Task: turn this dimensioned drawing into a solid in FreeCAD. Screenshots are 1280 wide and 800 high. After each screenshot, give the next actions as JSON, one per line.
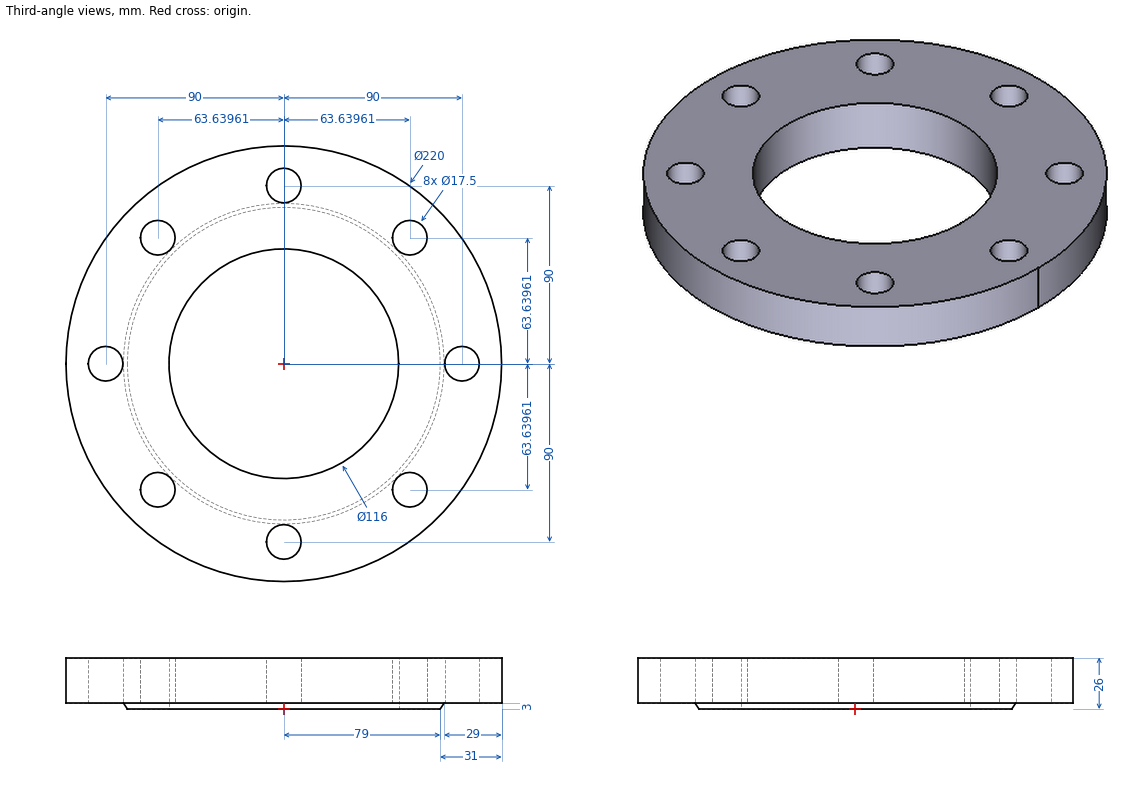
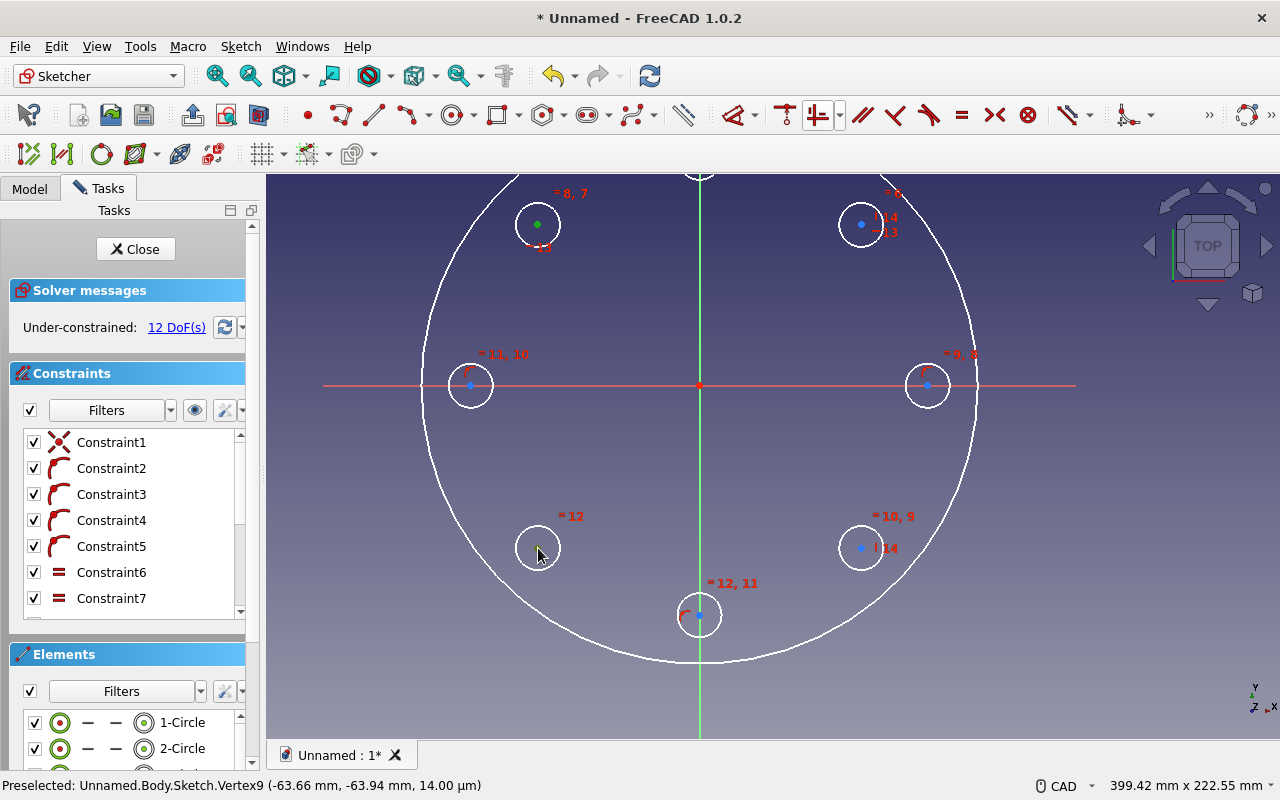
{"action": "left_click", "coordinate": [840, 116]}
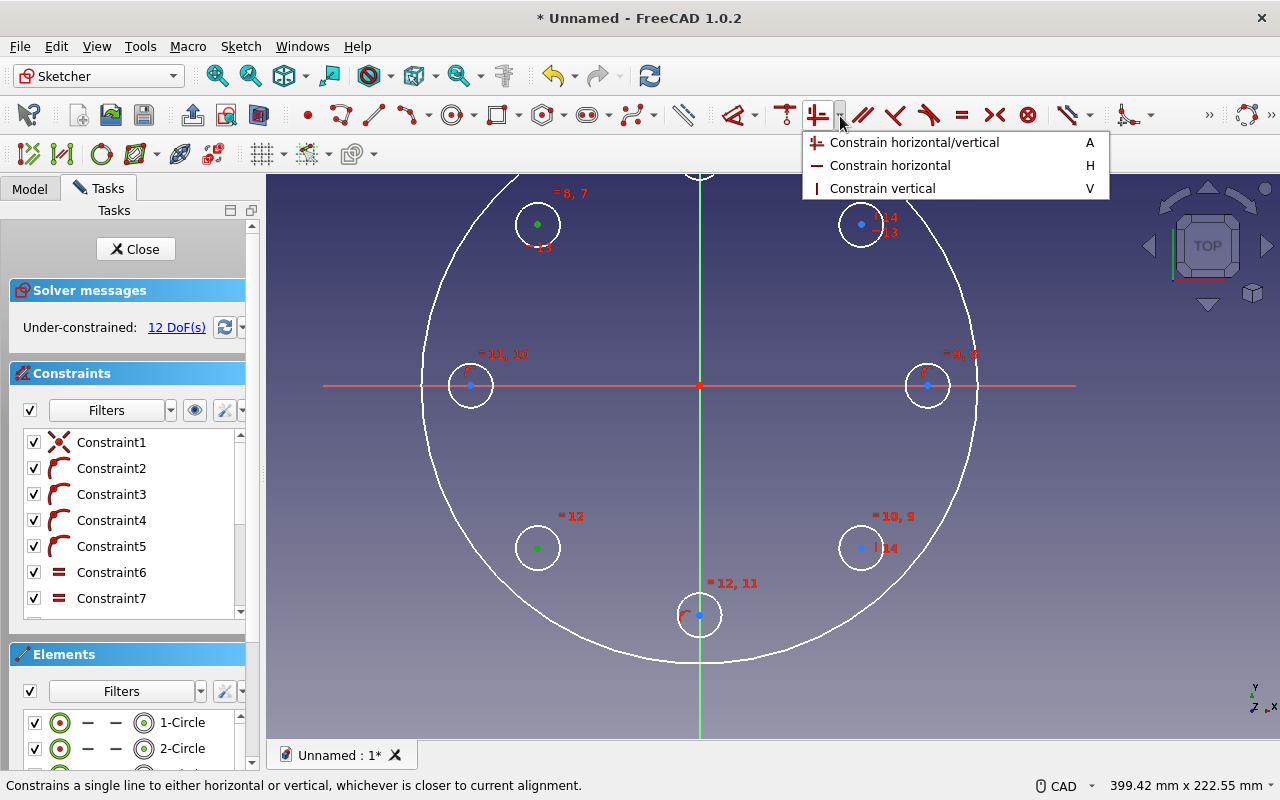
{"action": "left_click", "coordinate": [956, 188]}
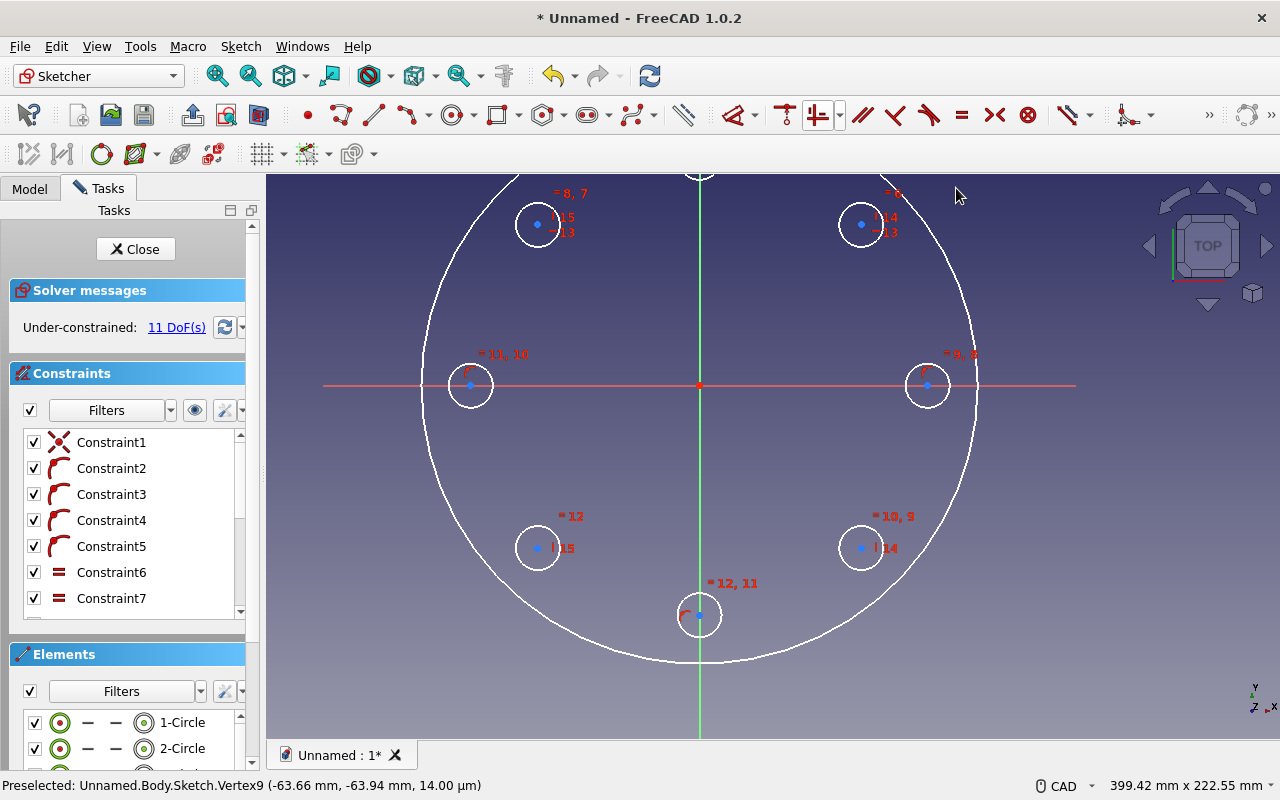
{"action": "left_click", "coordinate": [861, 548]}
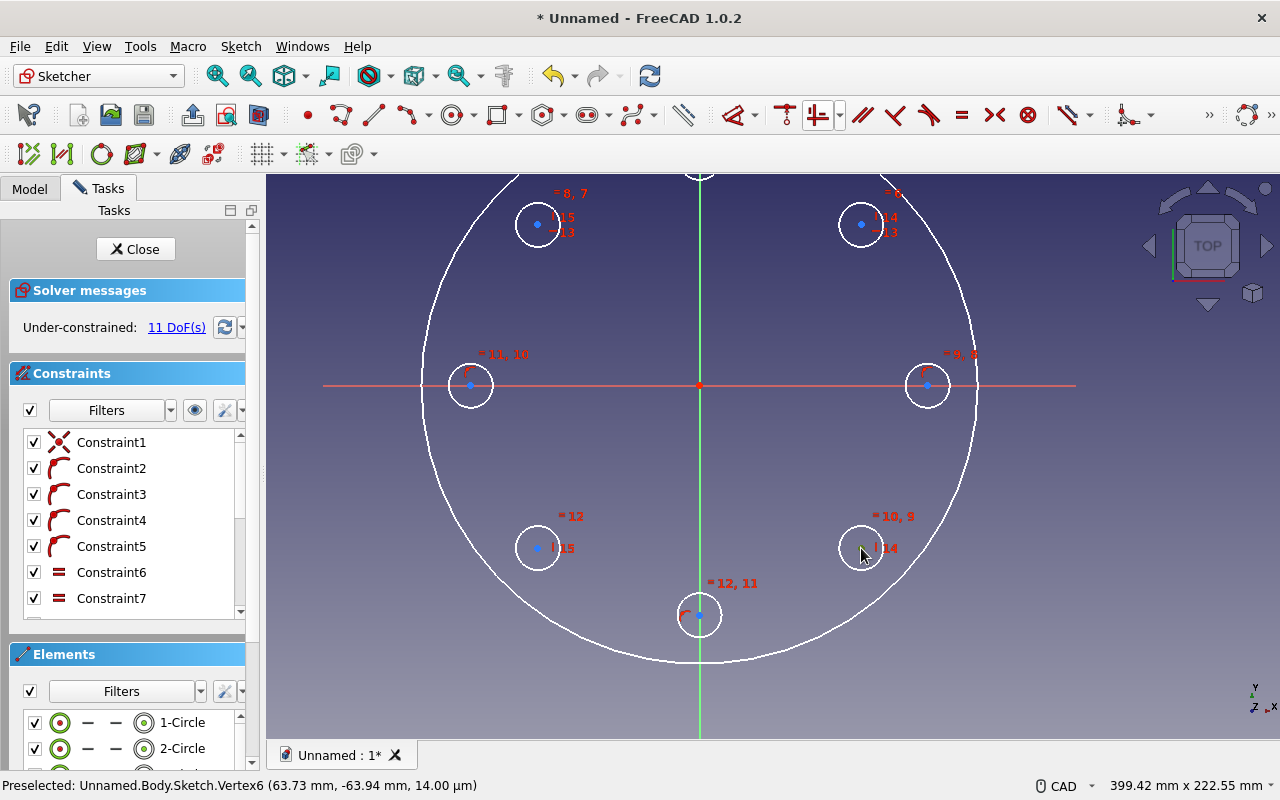
{"action": "left_click", "coordinate": [538, 548]}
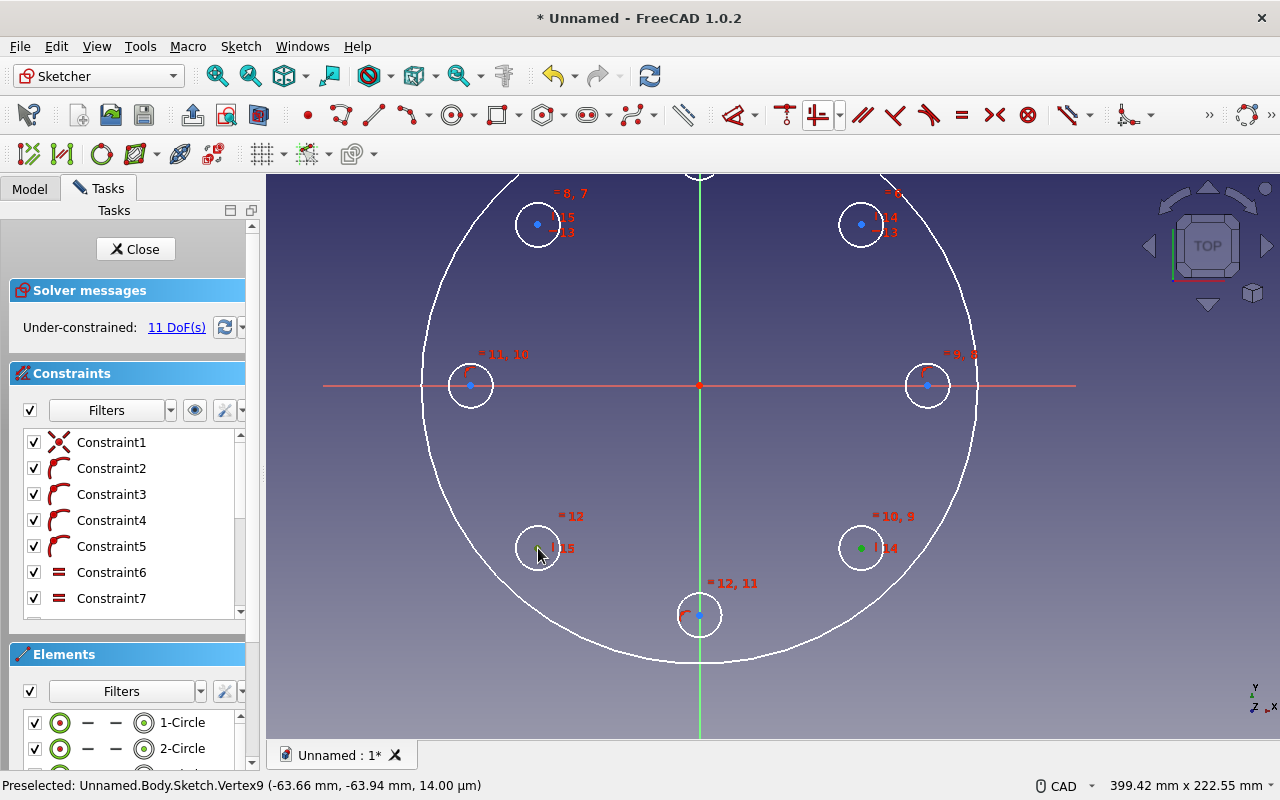
{"action": "left_click", "coordinate": [840, 116]}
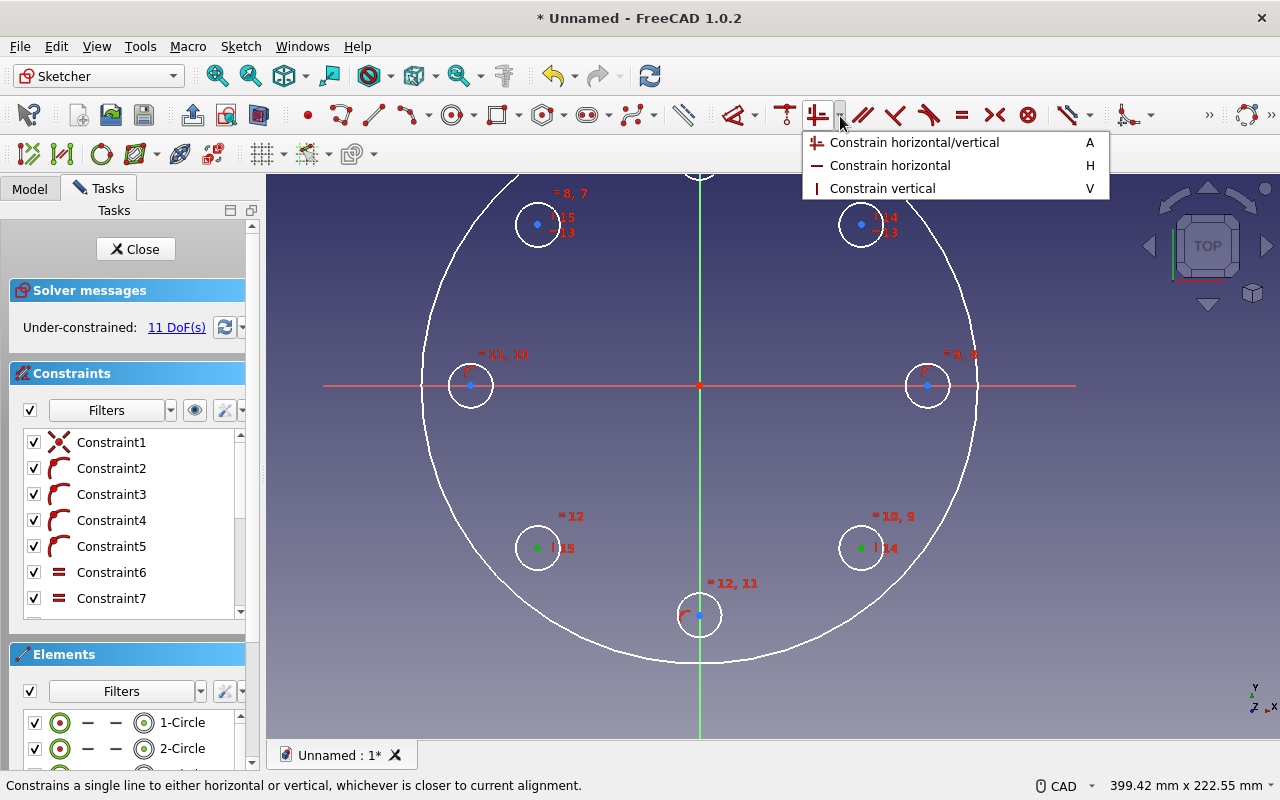
{"action": "left_click", "coordinate": [956, 166]}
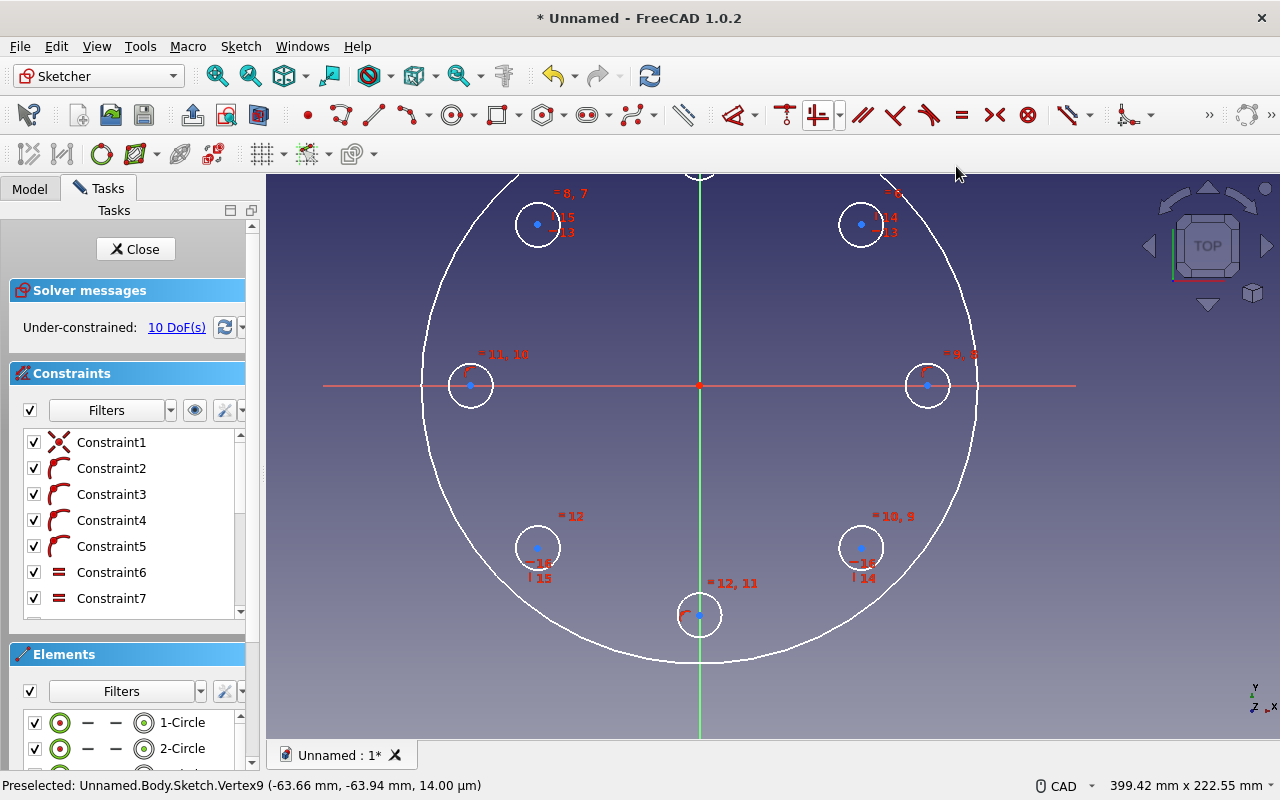
{"action": "left_click", "coordinate": [503, 583]}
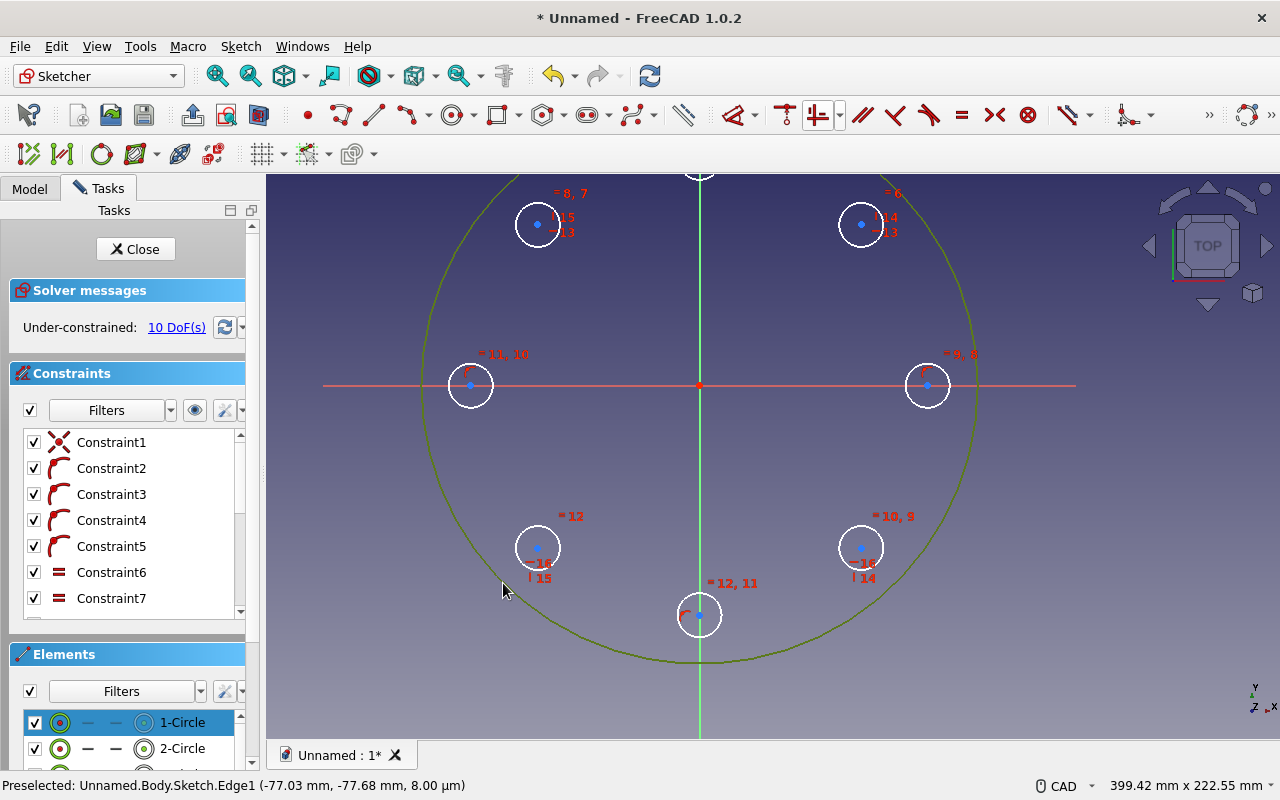
{"action": "key", "text": "k o"}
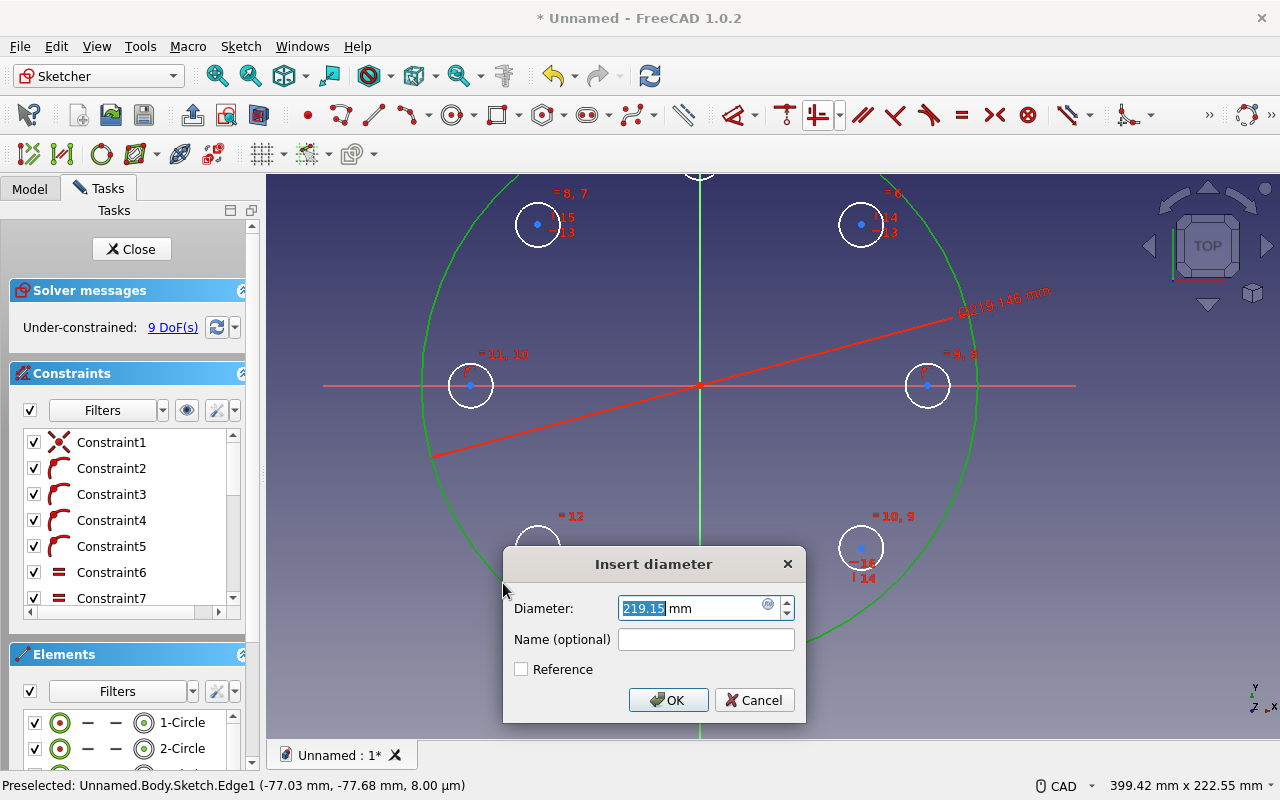
{"action": "type", "text": "220"}
{"action": "key", "text": "Return"}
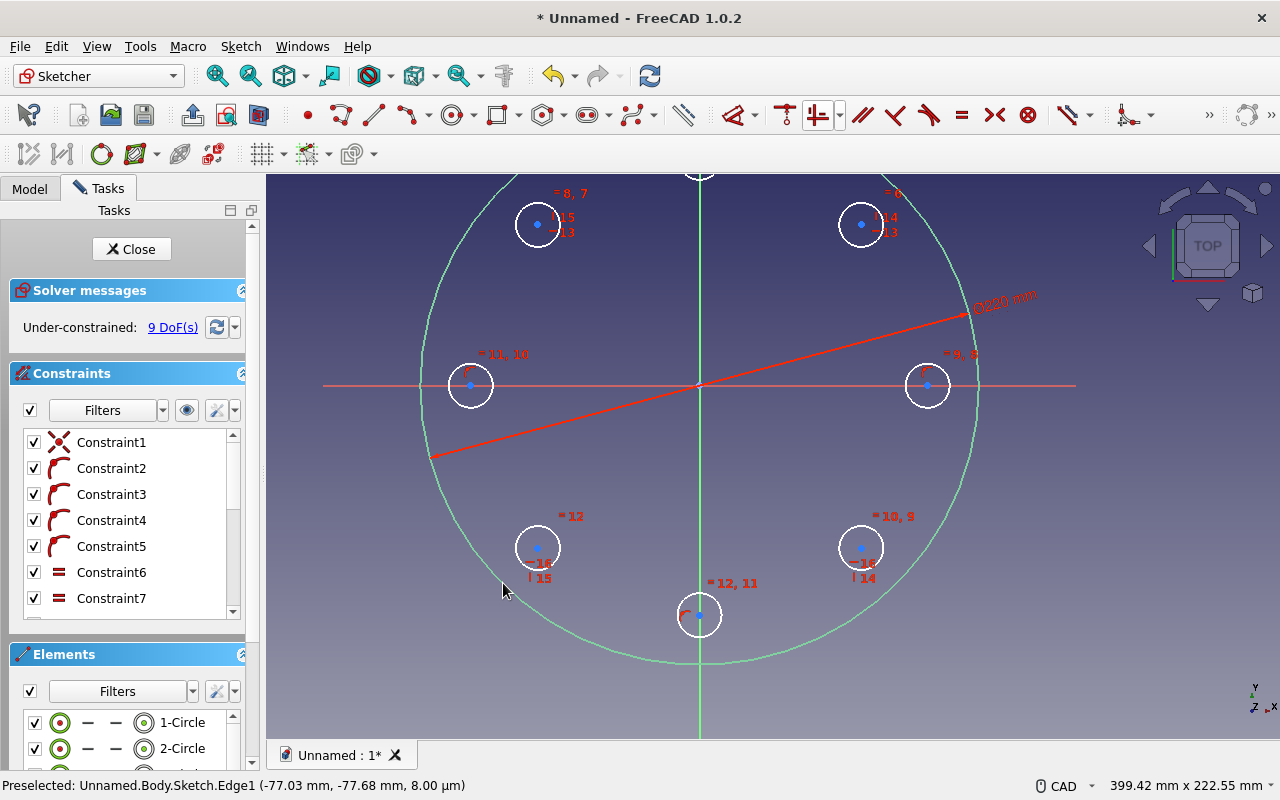
{"action": "left_click", "coordinate": [846, 209]}